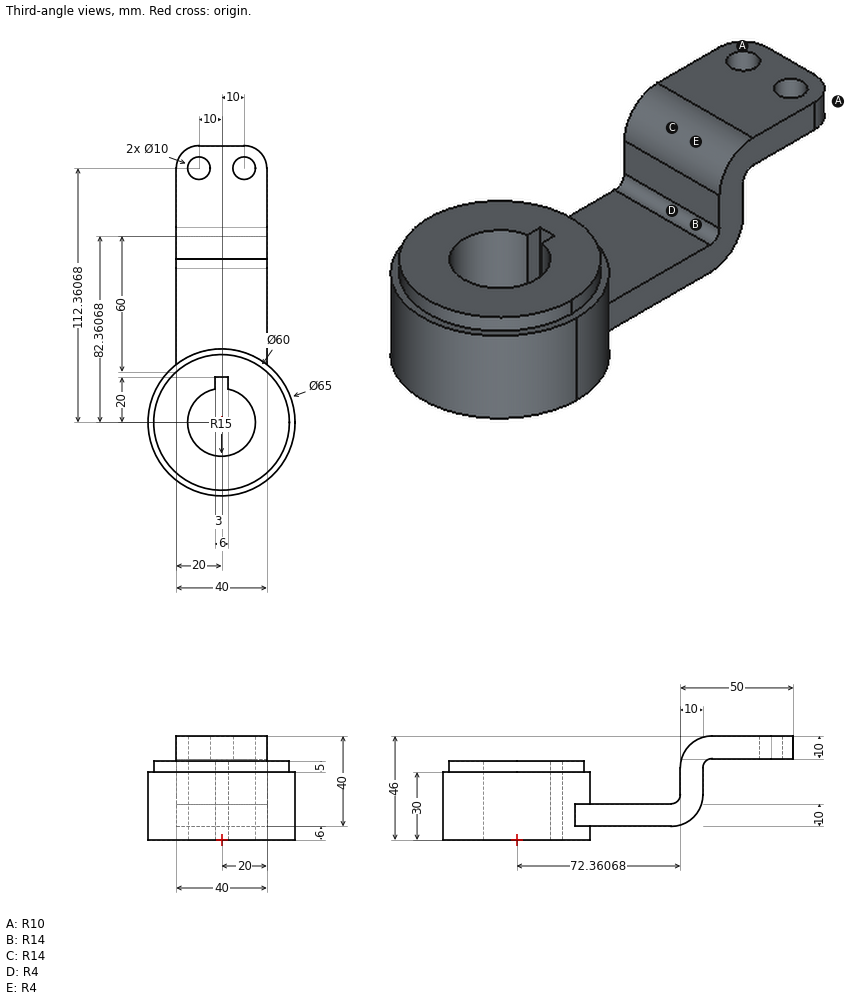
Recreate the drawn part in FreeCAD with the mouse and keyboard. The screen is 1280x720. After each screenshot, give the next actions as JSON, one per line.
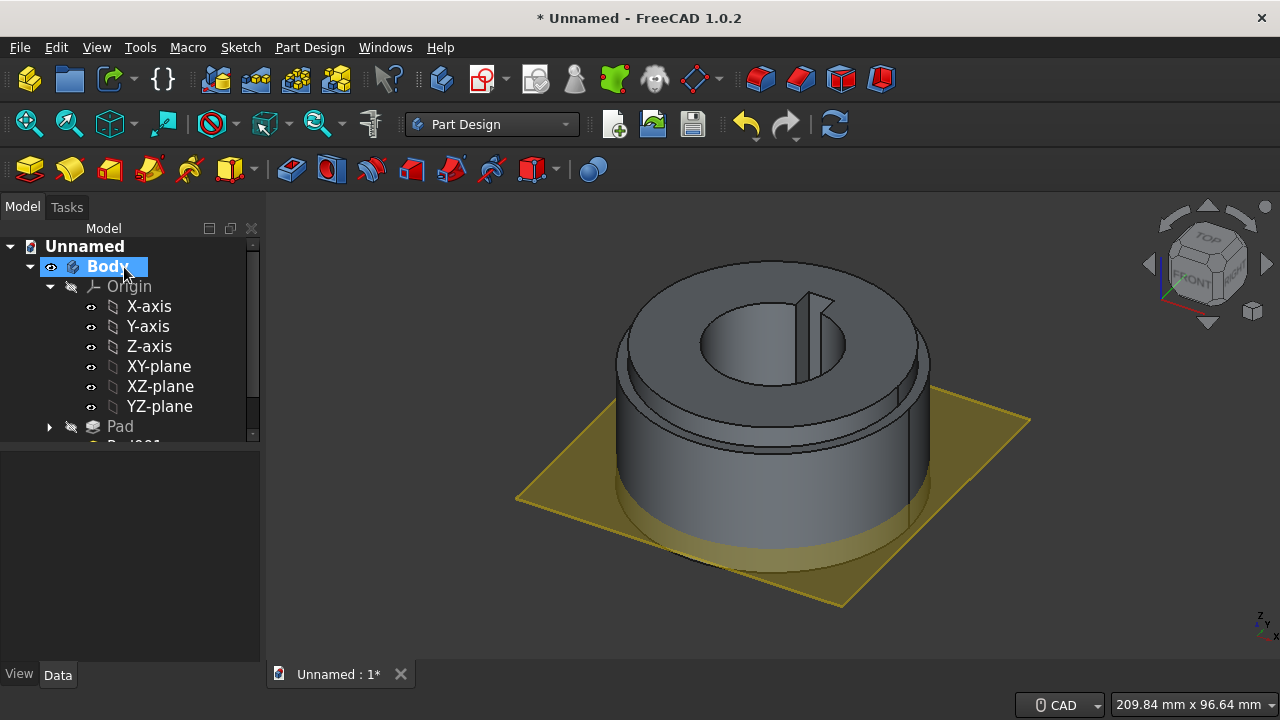
{"action": "scroll", "coordinate": [100, 342], "scroll_direction": "down", "scroll_amount": 3}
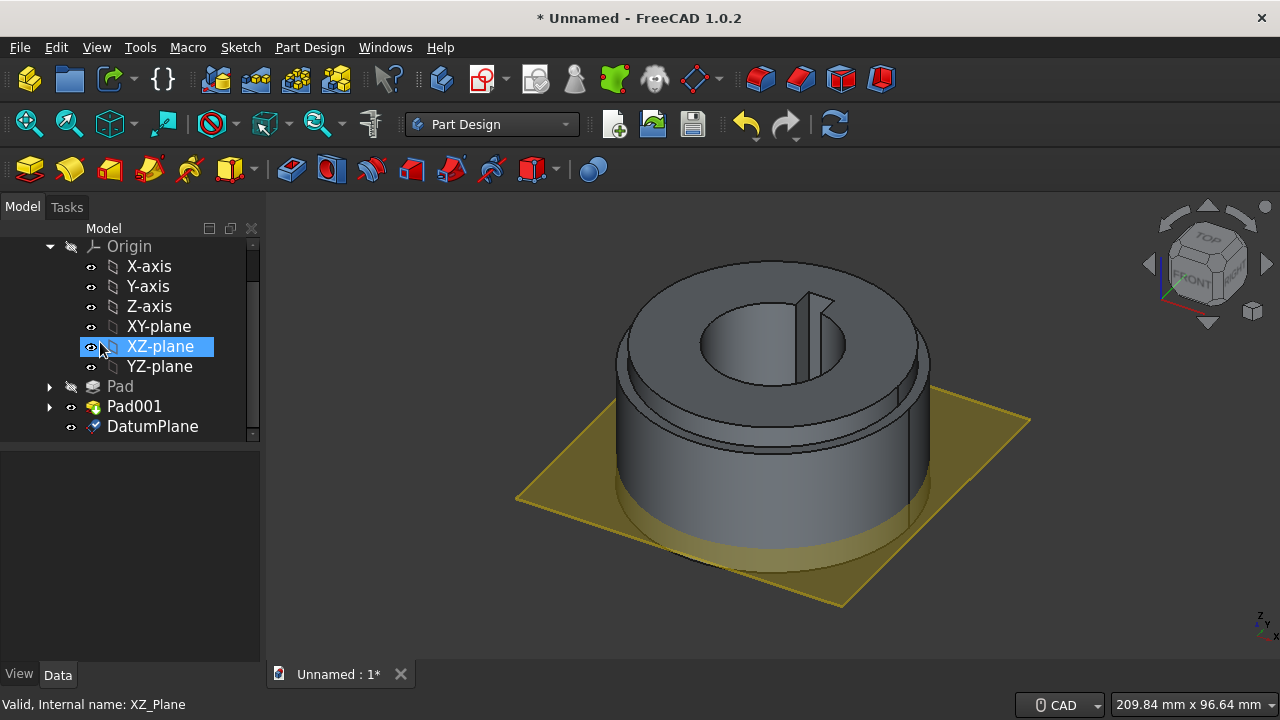
{"action": "left_click", "coordinate": [116, 427]}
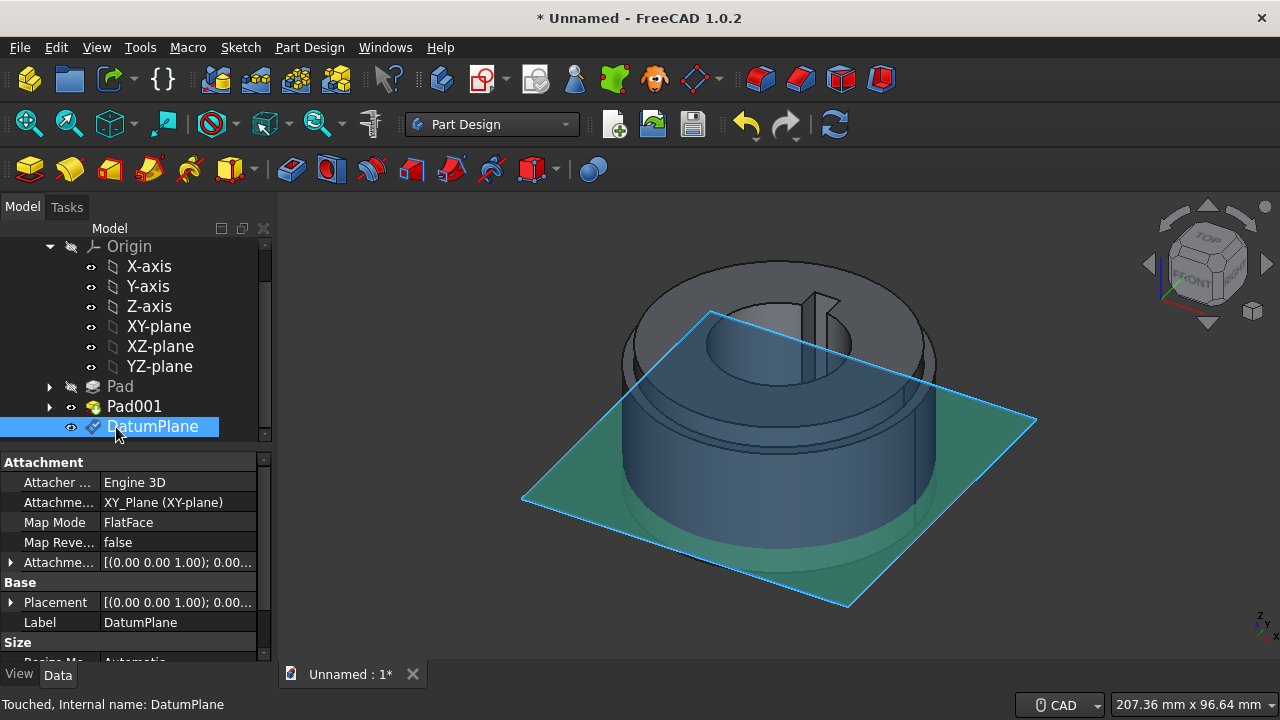
{"action": "left_click", "coordinate": [482, 80]}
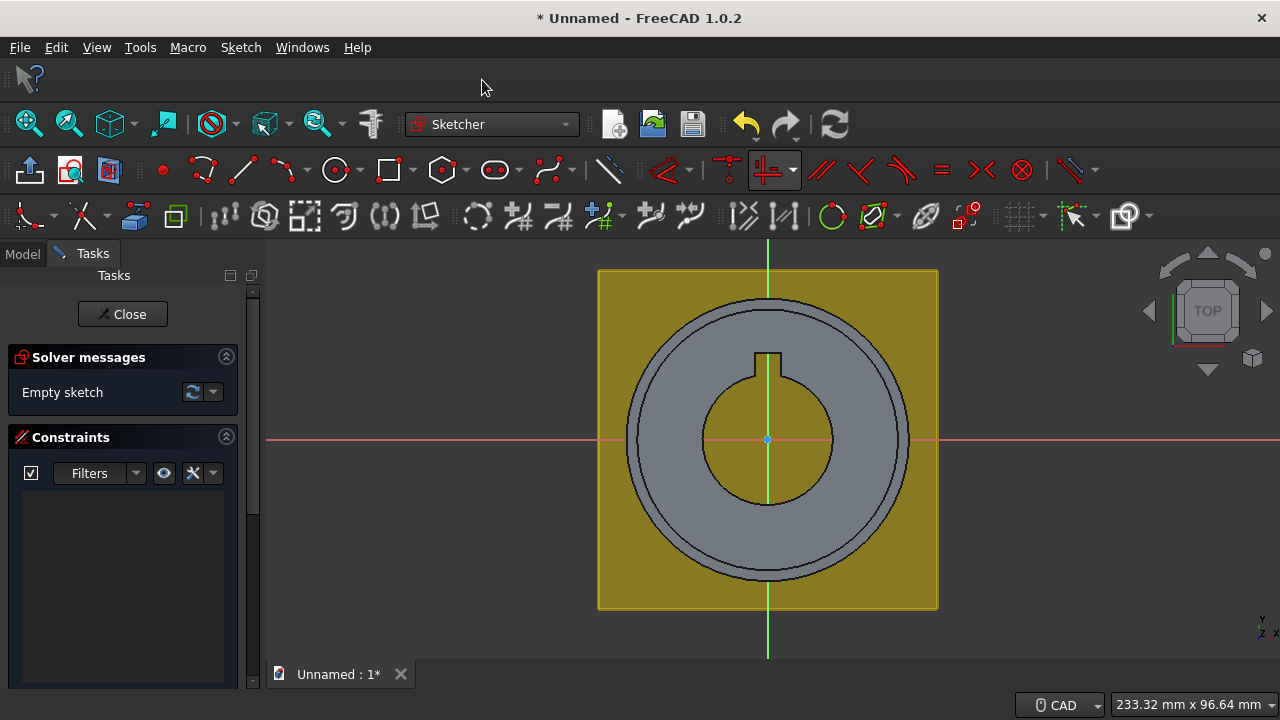
{"action": "left_click", "coordinate": [110, 170]}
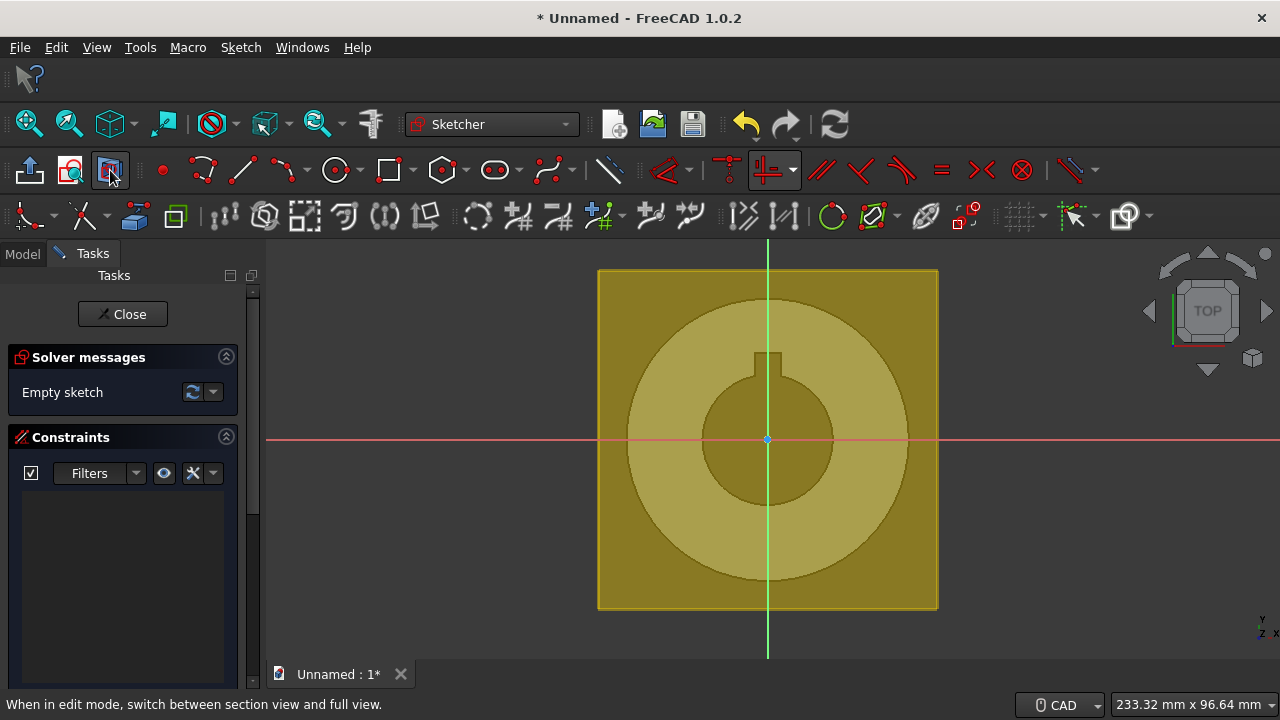
{"action": "scroll", "coordinate": [628, 631], "scroll_direction": "down", "scroll_amount": 3}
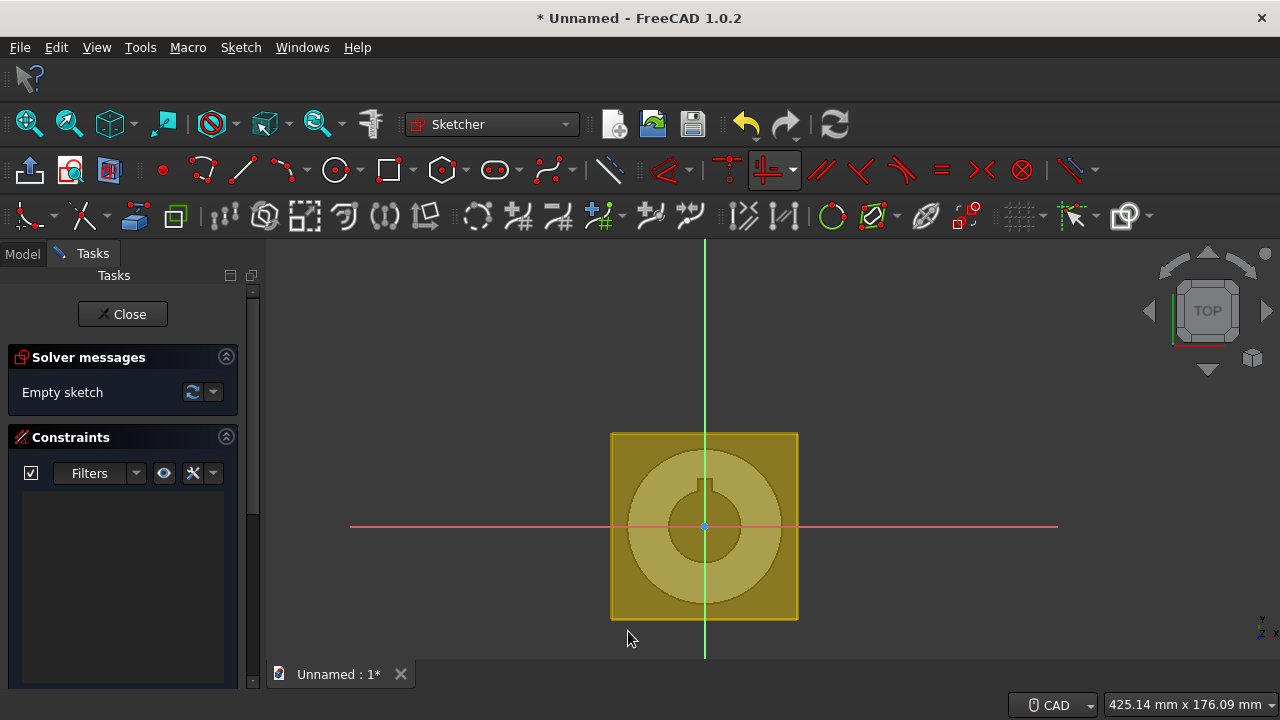
{"action": "key", "text": "g r"}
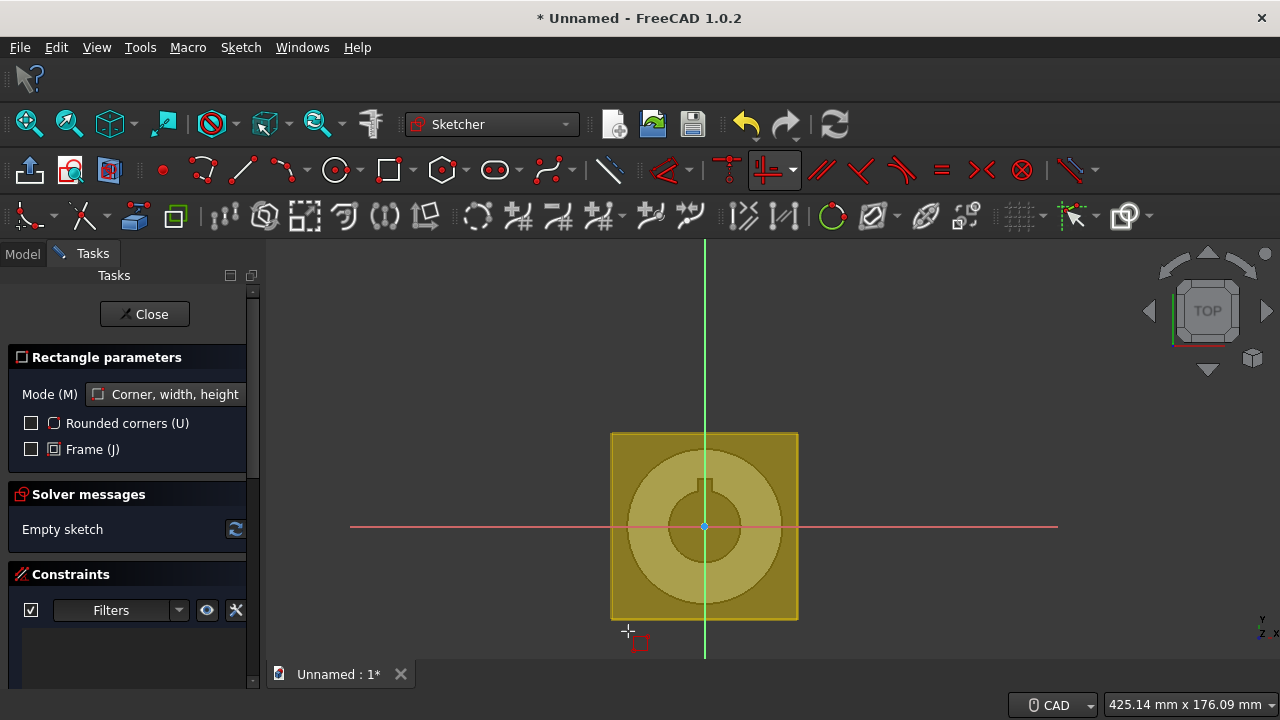
{"action": "left_click", "coordinate": [657, 330]}
{"action": "left_click", "coordinate": [752, 473]}
{"action": "key", "text": "Escape"}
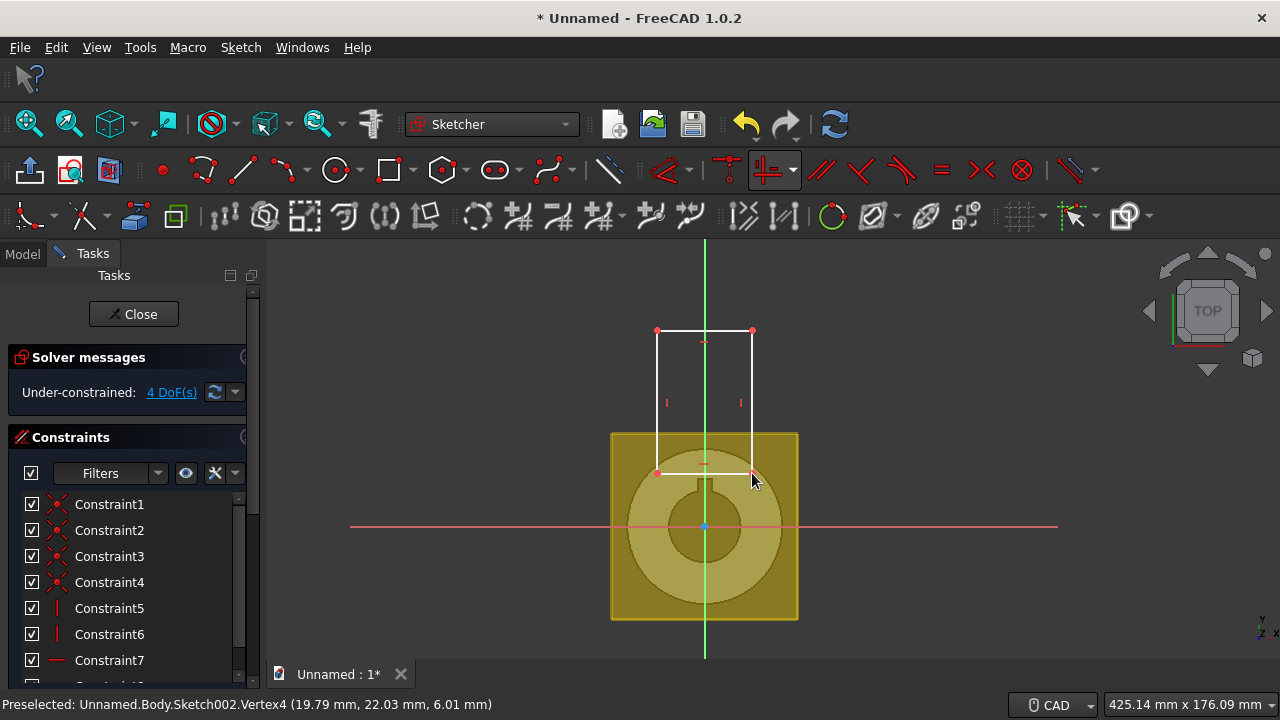
{"action": "key", "text": "d"}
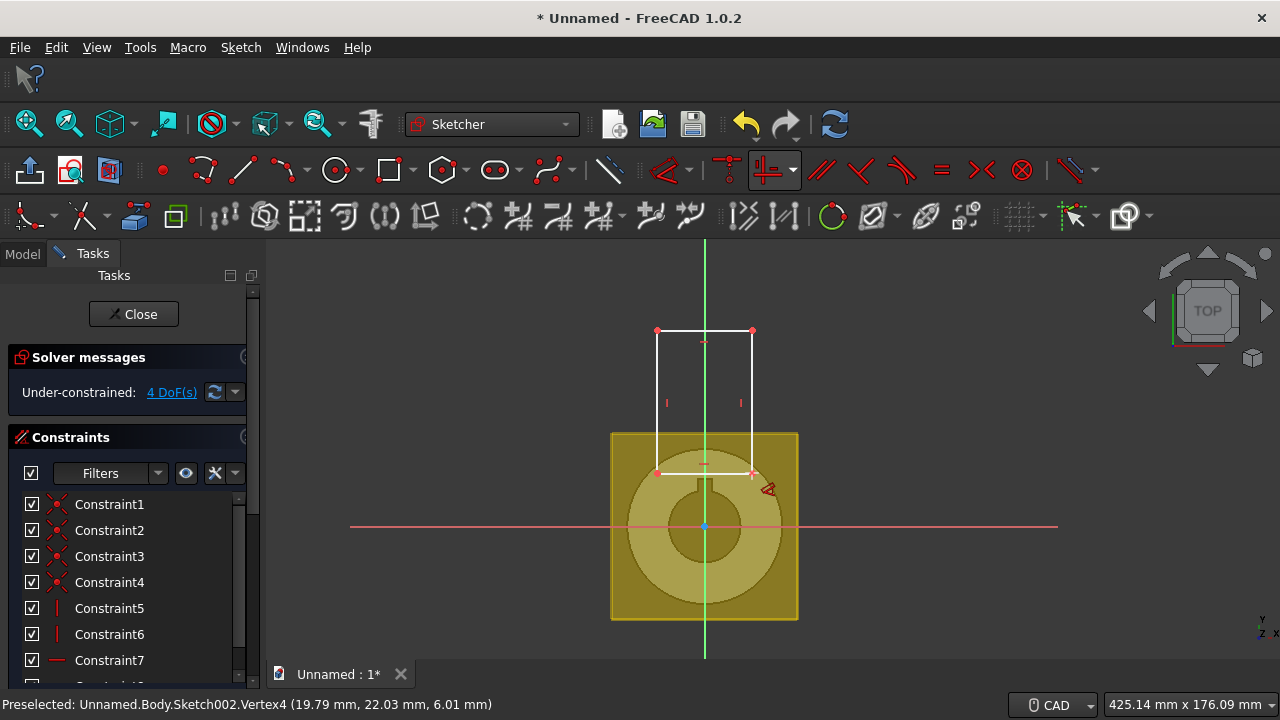
{"action": "left_click", "coordinate": [657, 374]}
{"action": "left_click", "coordinate": [623, 402]}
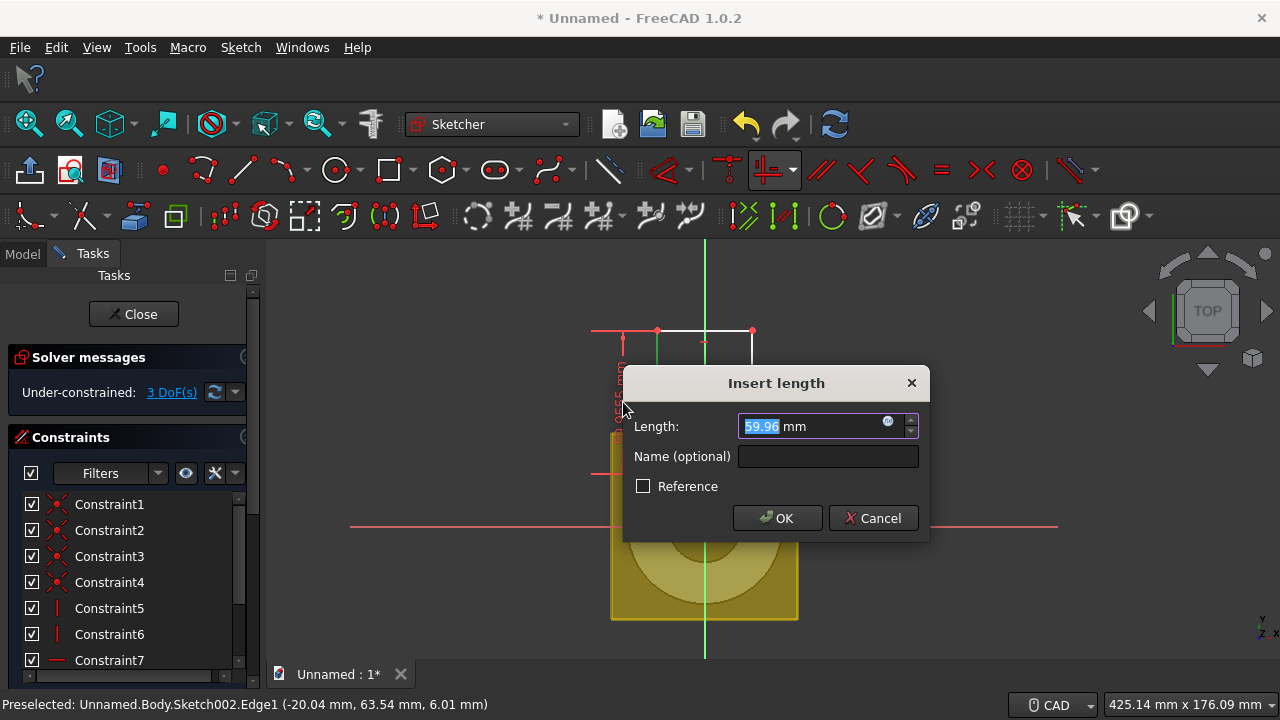
{"action": "type", "text": "60"}
{"action": "key", "text": "Return"}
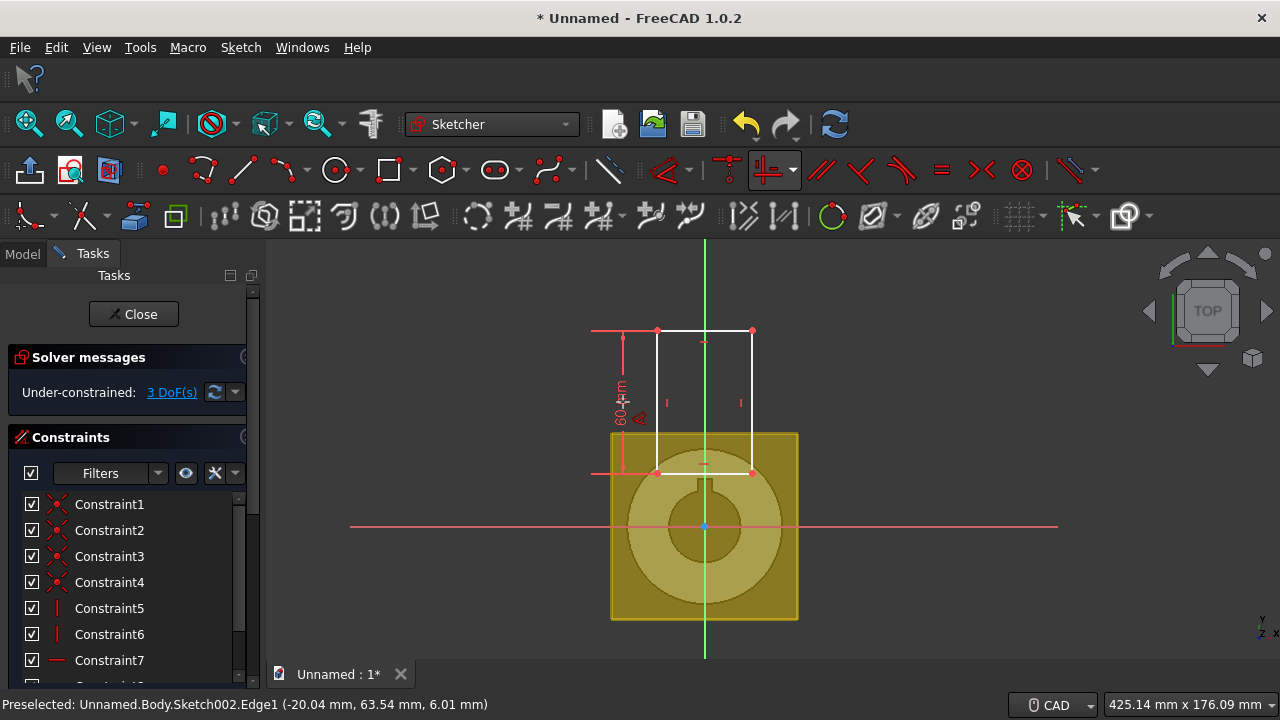
{"action": "left_click", "coordinate": [686, 474]}
{"action": "left_click", "coordinate": [683, 508]}